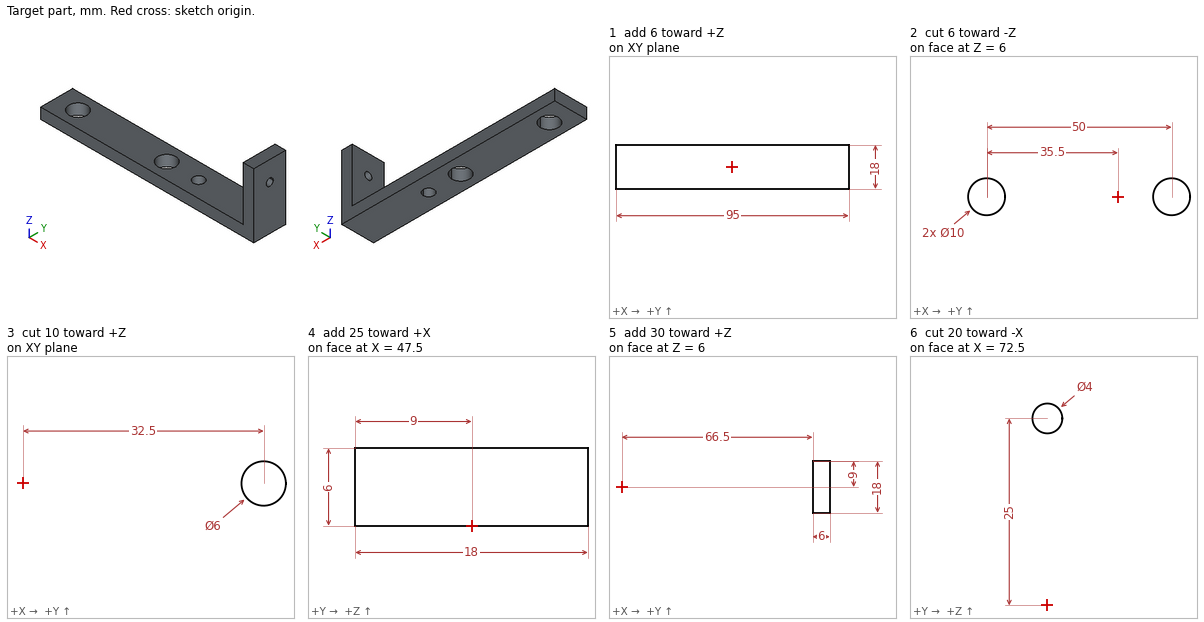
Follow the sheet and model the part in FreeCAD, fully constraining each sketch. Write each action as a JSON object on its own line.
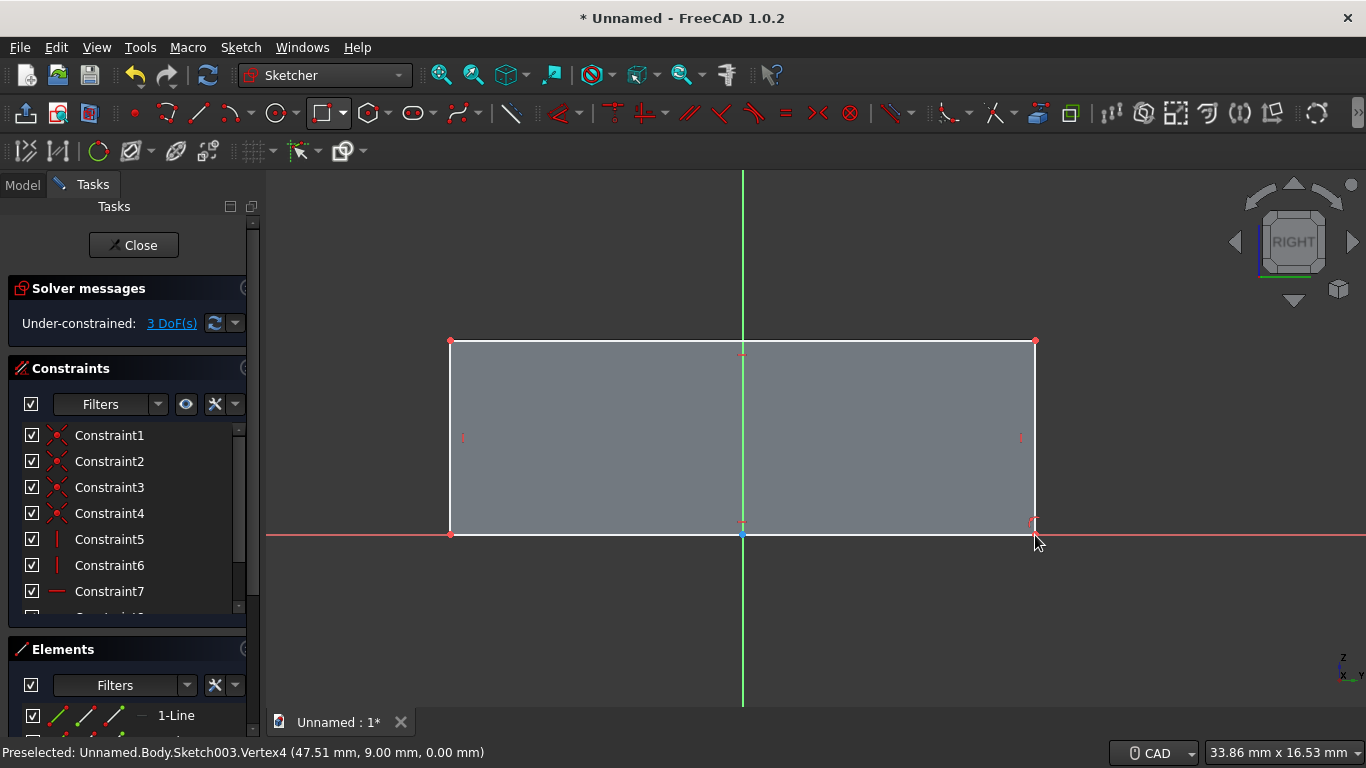
{"action": "left_click", "coordinate": [558, 114]}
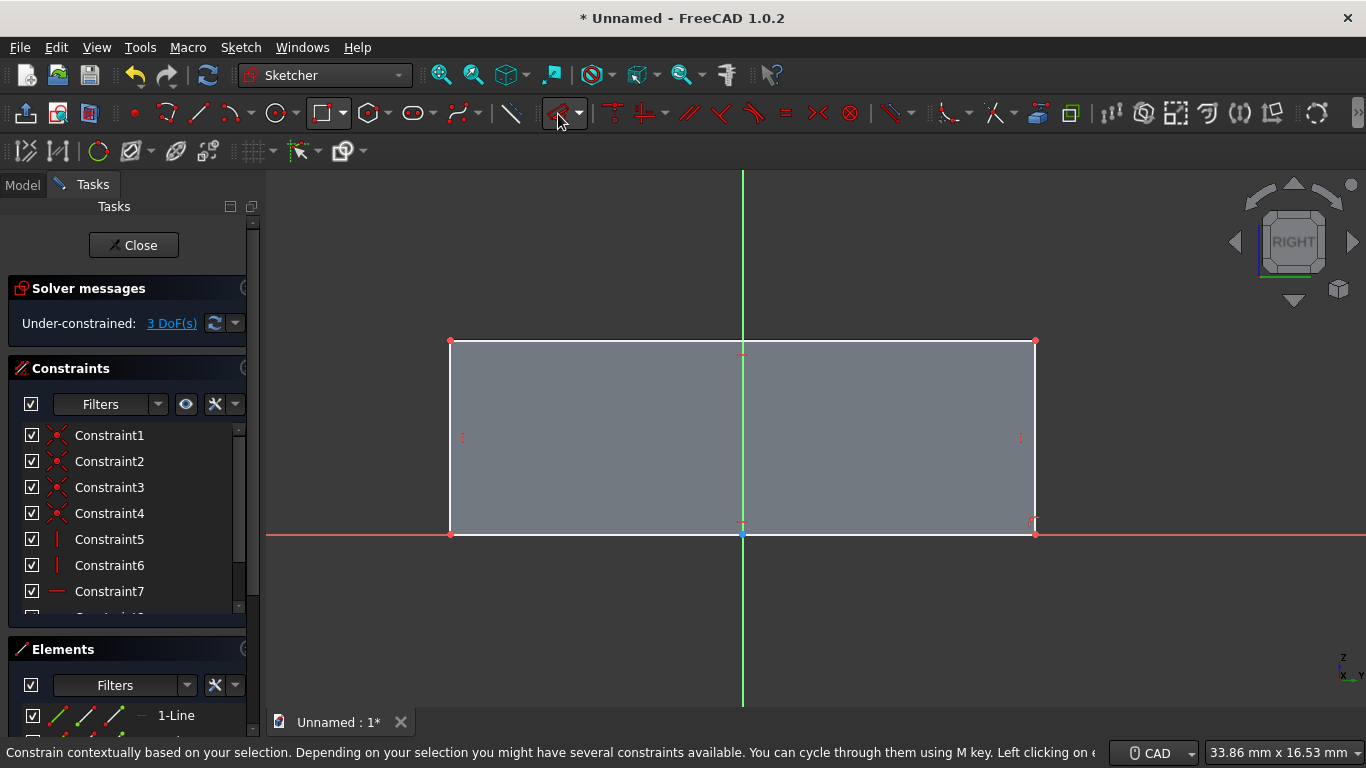
{"action": "left_click", "coordinate": [450, 399]}
{"action": "left_click", "coordinate": [416, 438]}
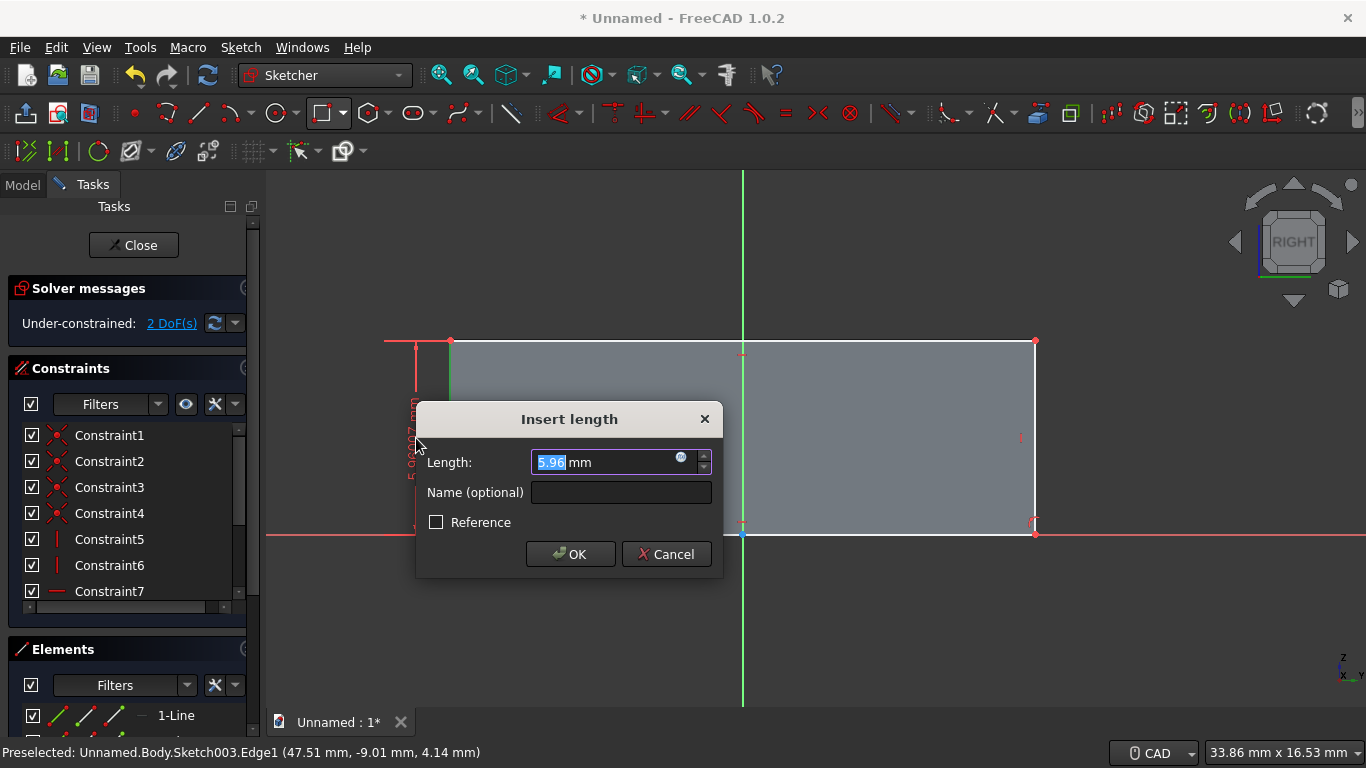
{"action": "type", "text": "6"}
{"action": "key", "text": "Return"}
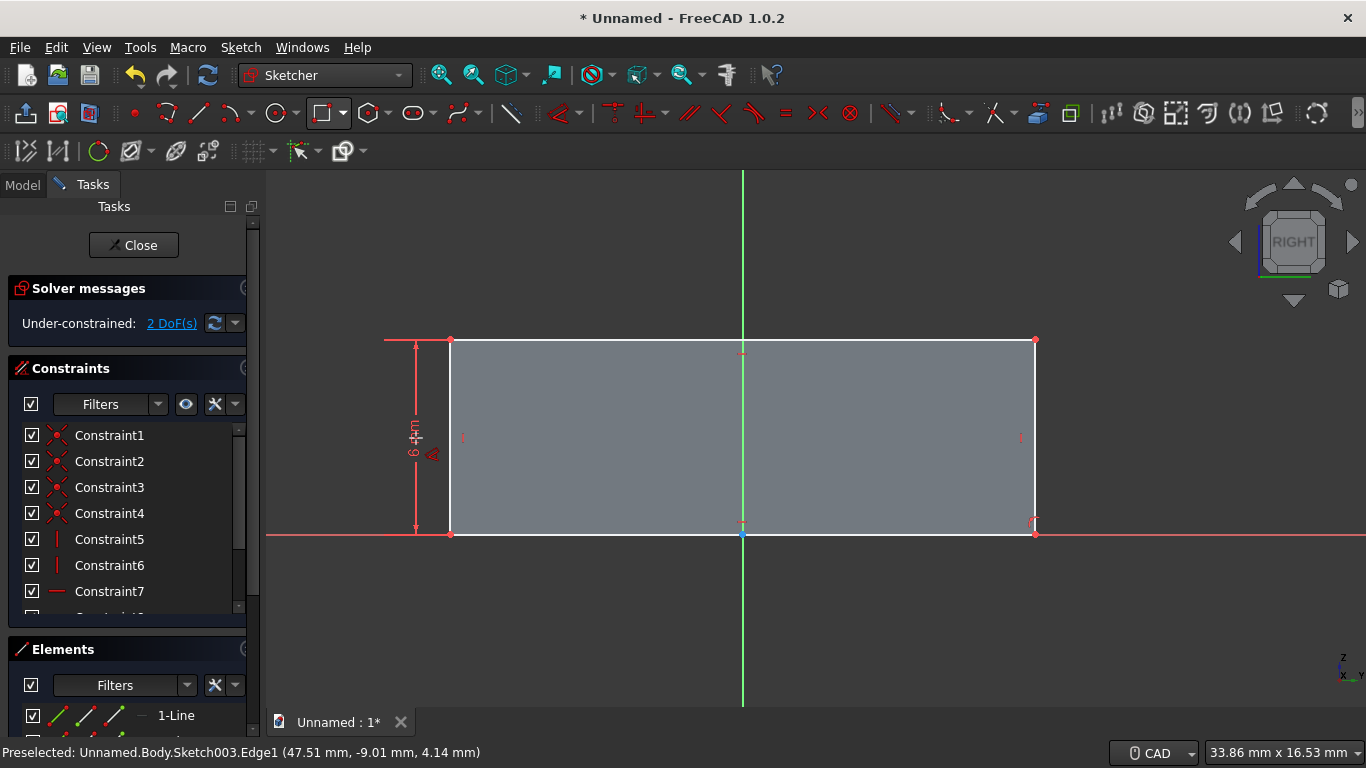
{"action": "left_click", "coordinate": [626, 535]}
{"action": "left_click", "coordinate": [608, 569]}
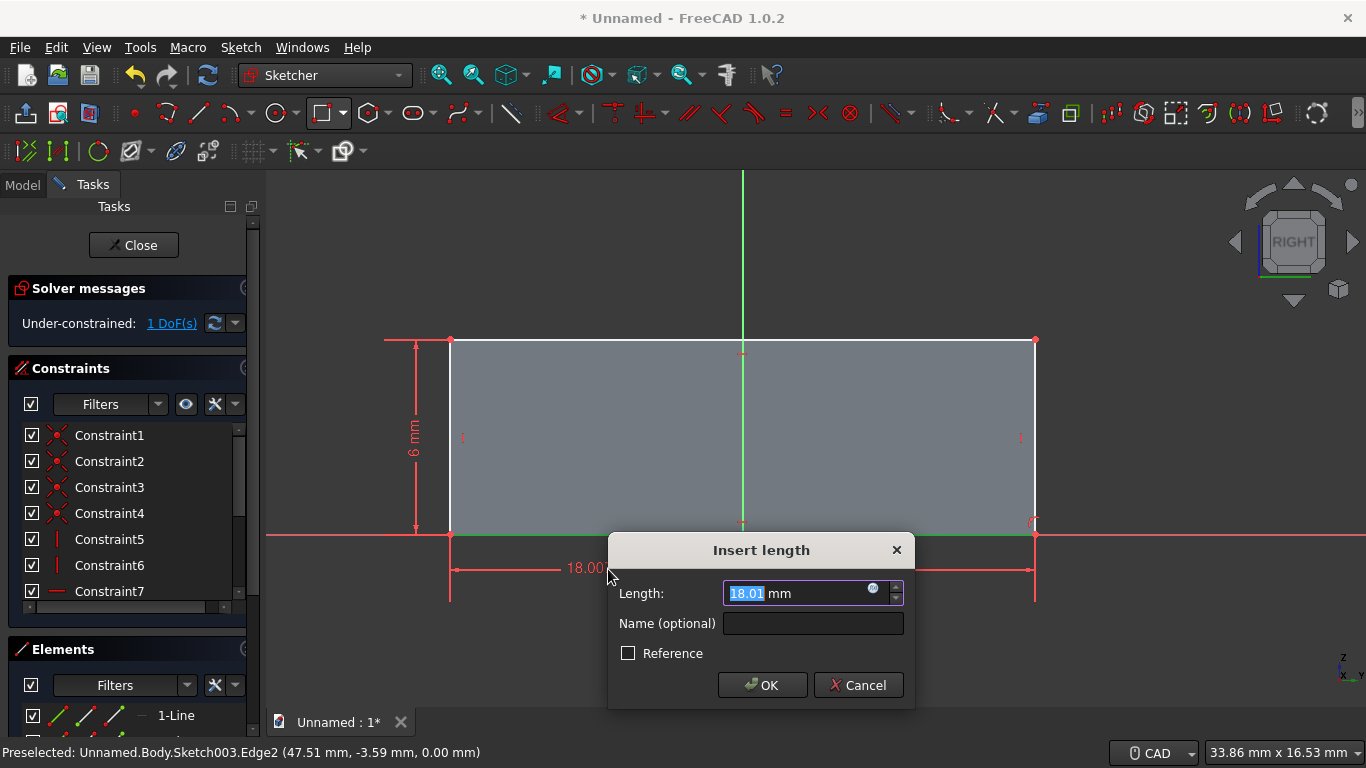
{"action": "type", "text": "18"}
{"action": "key", "text": "Return"}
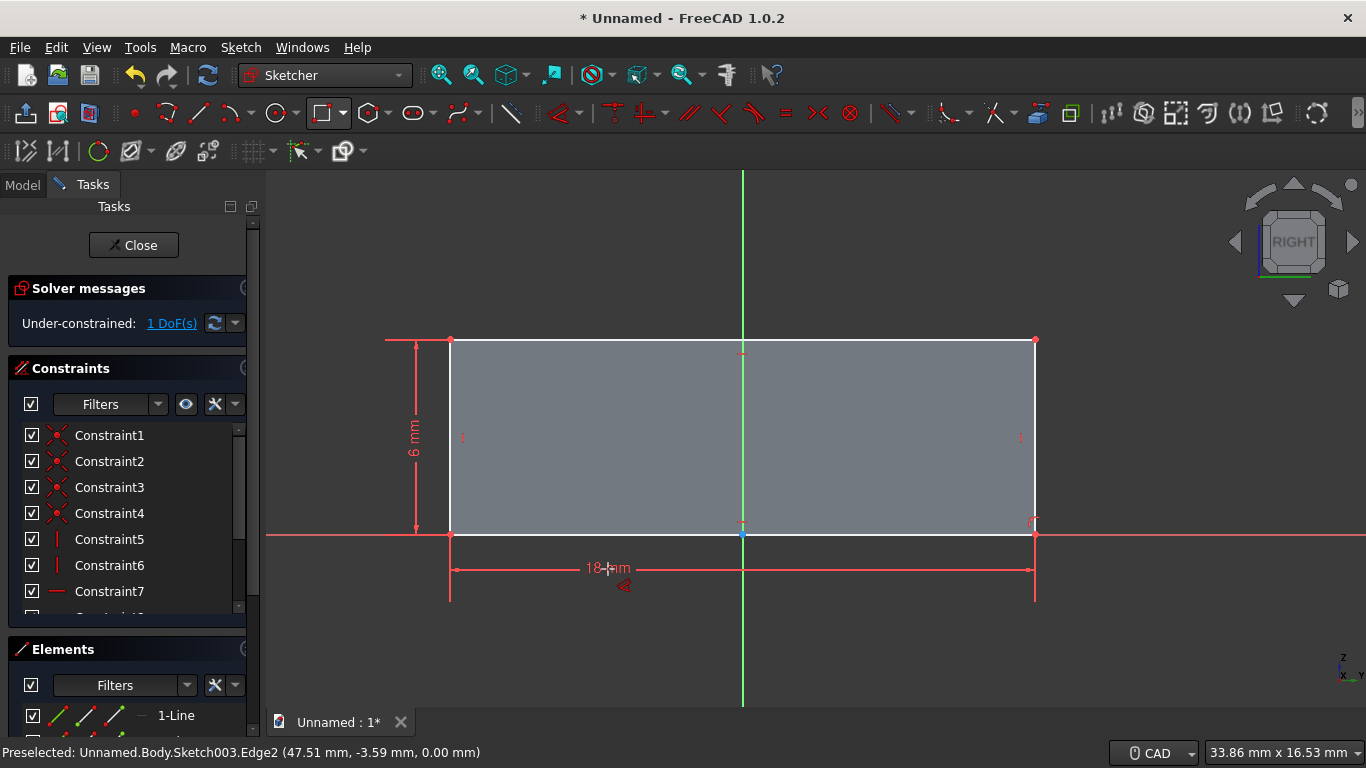
{"action": "left_click", "coordinate": [450, 340]}
{"action": "left_click", "coordinate": [529, 569]}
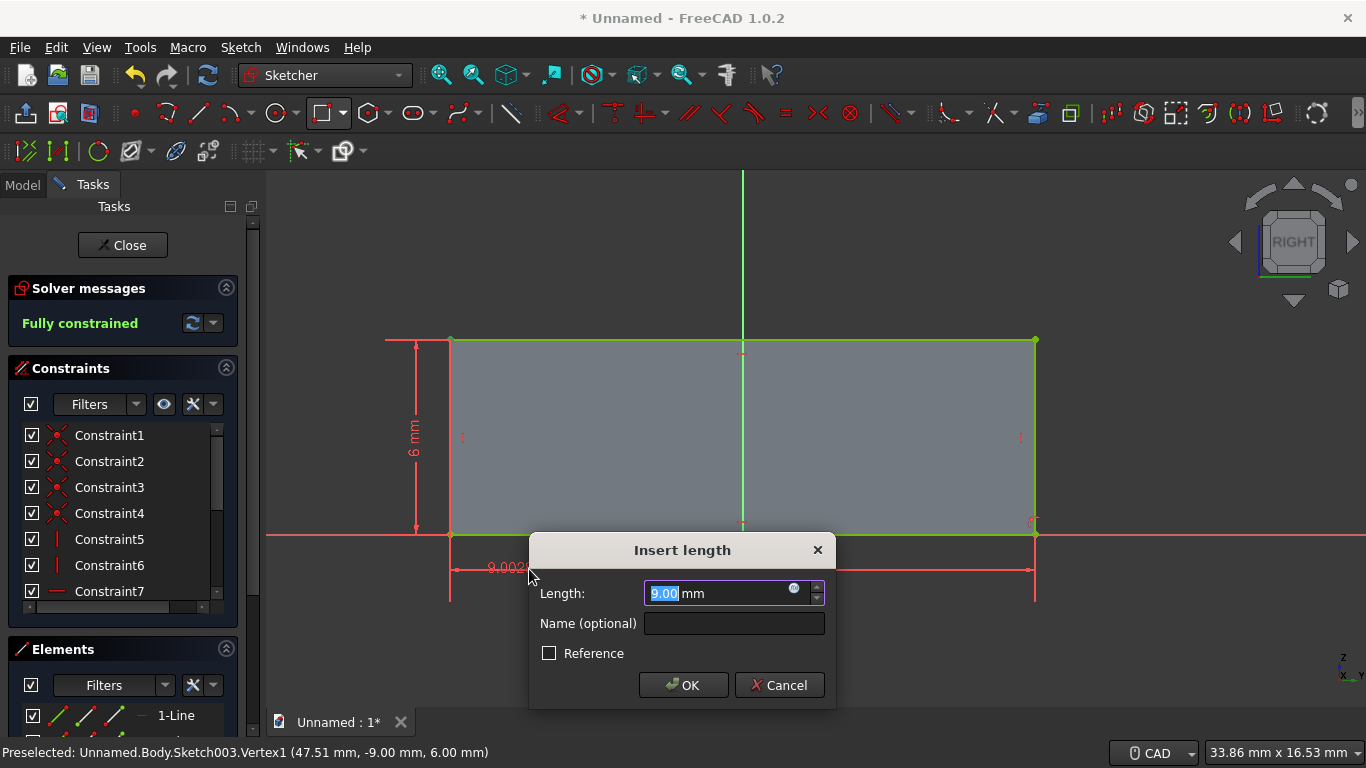
{"action": "type", "text": "9"}
{"action": "key", "text": "Return"}
{"action": "key", "text": "Escape"}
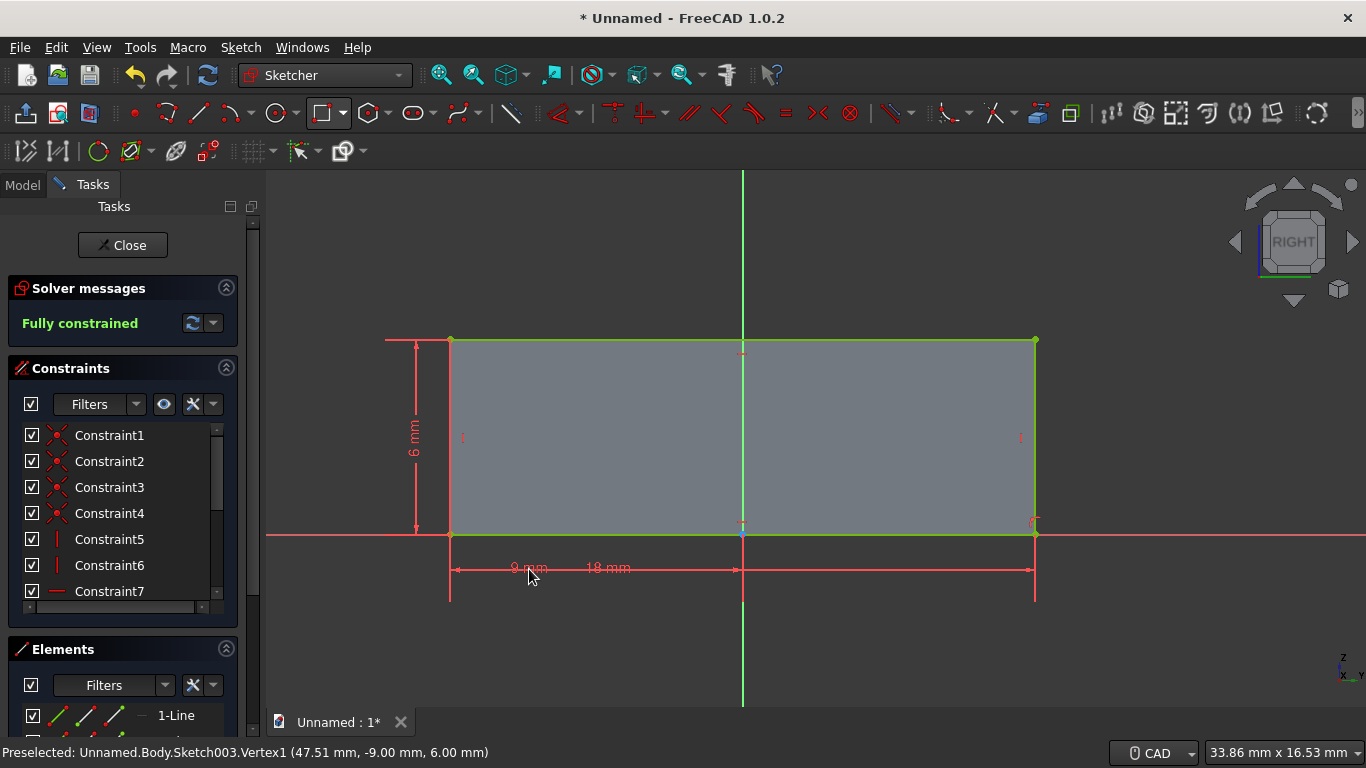
{"action": "left_click", "coordinate": [123, 245]}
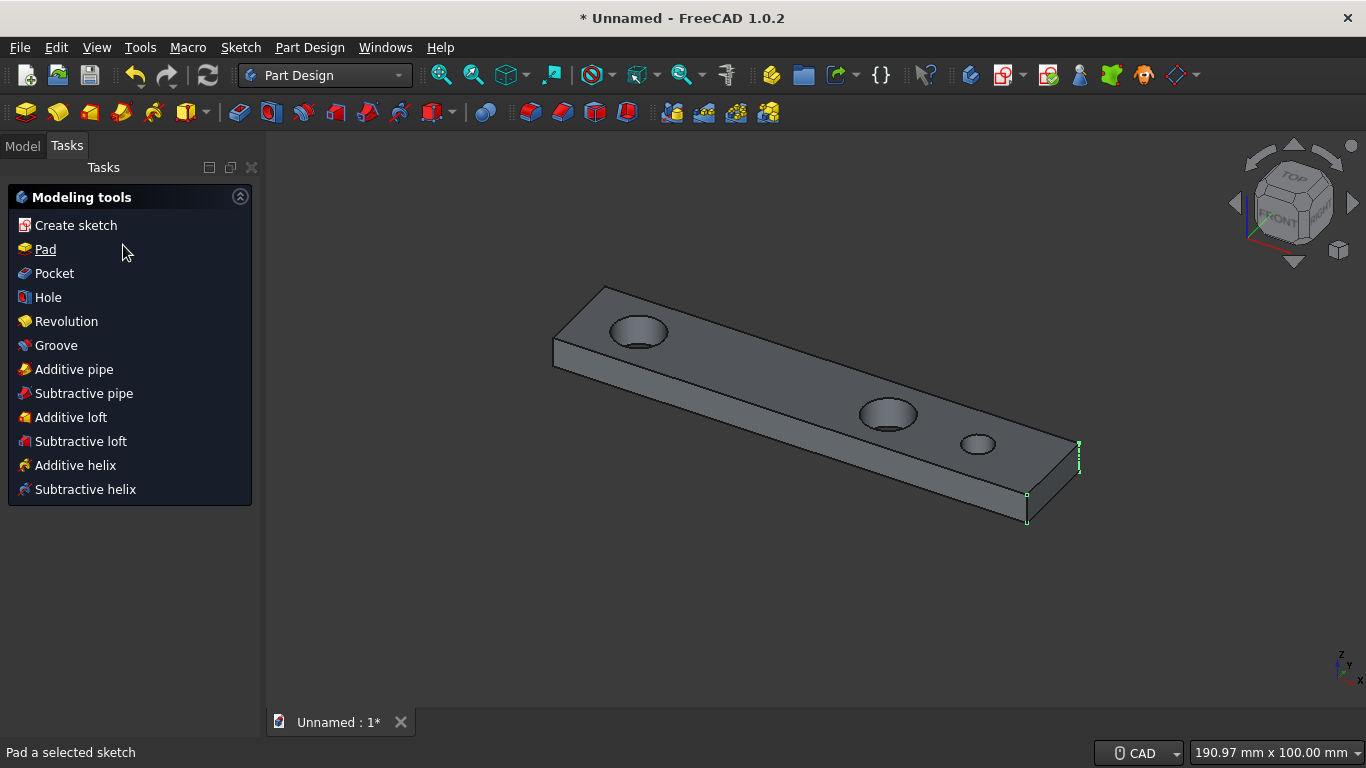
{"action": "left_click", "coordinate": [26, 112]}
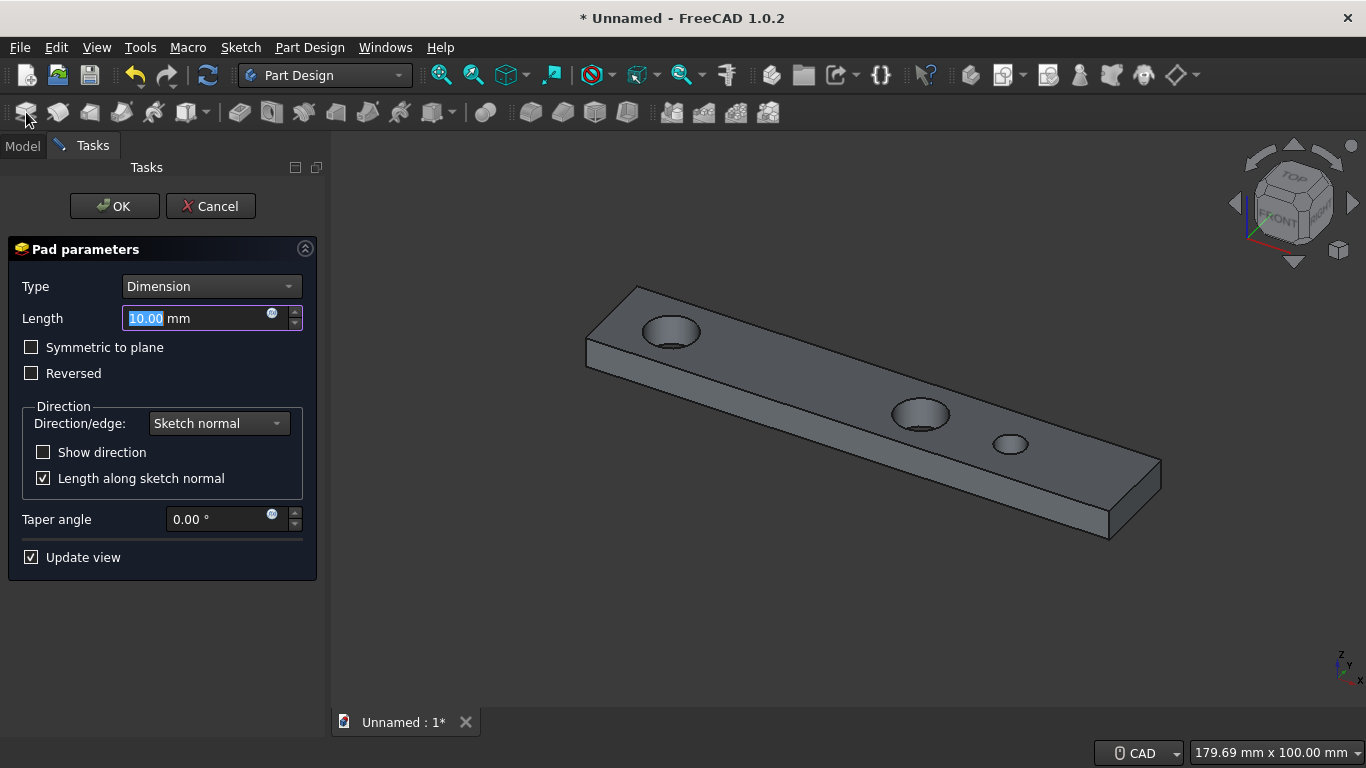
{"action": "type", "text": "25"}
{"action": "key", "text": "Tab"}